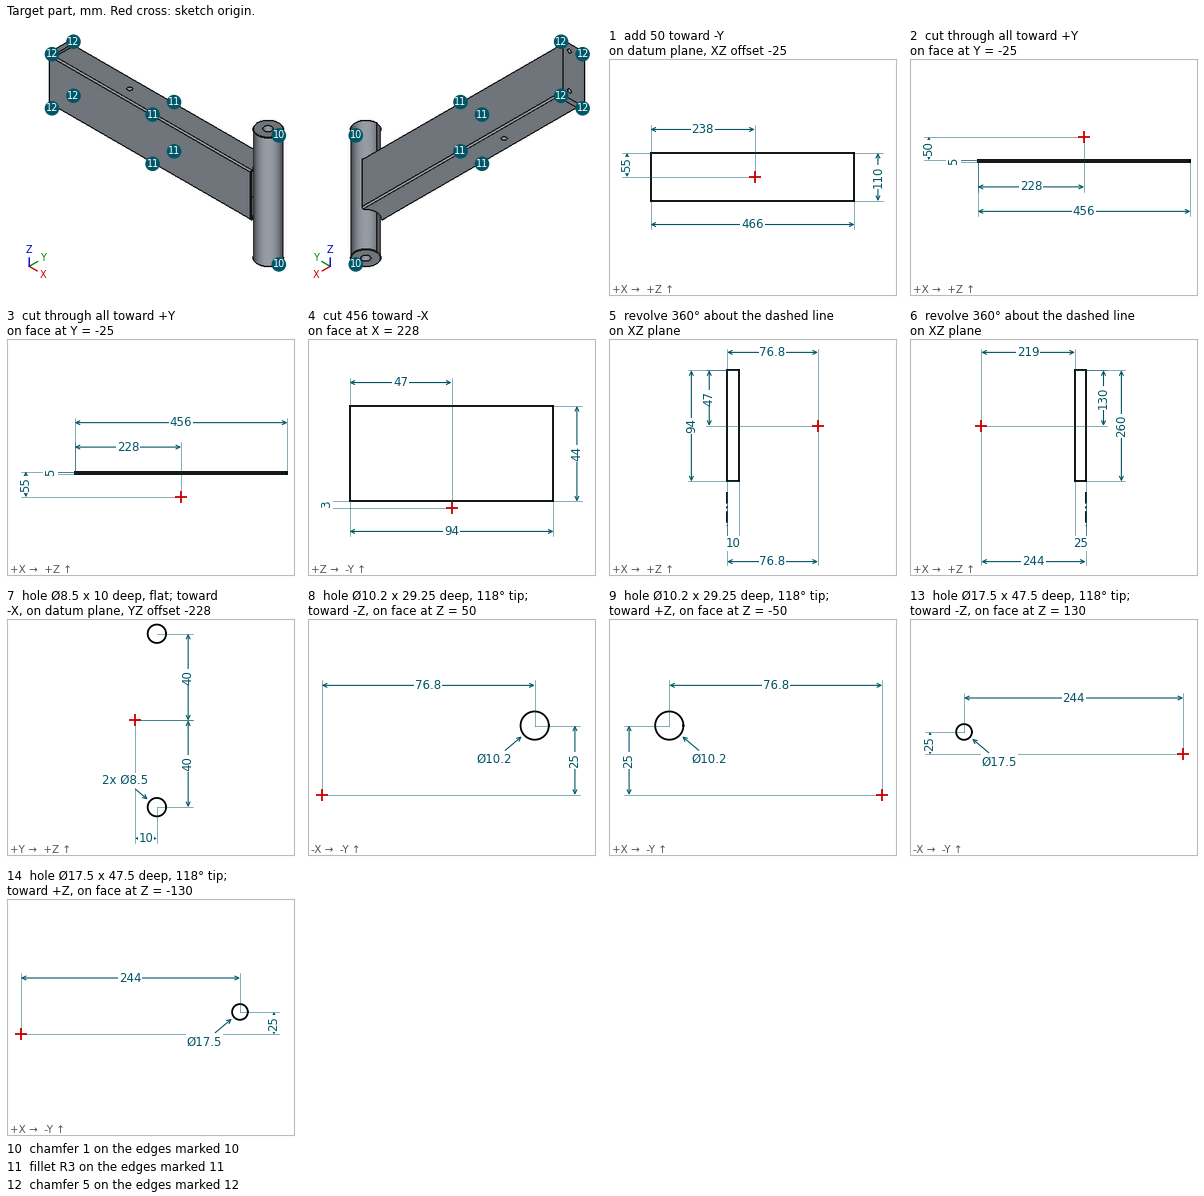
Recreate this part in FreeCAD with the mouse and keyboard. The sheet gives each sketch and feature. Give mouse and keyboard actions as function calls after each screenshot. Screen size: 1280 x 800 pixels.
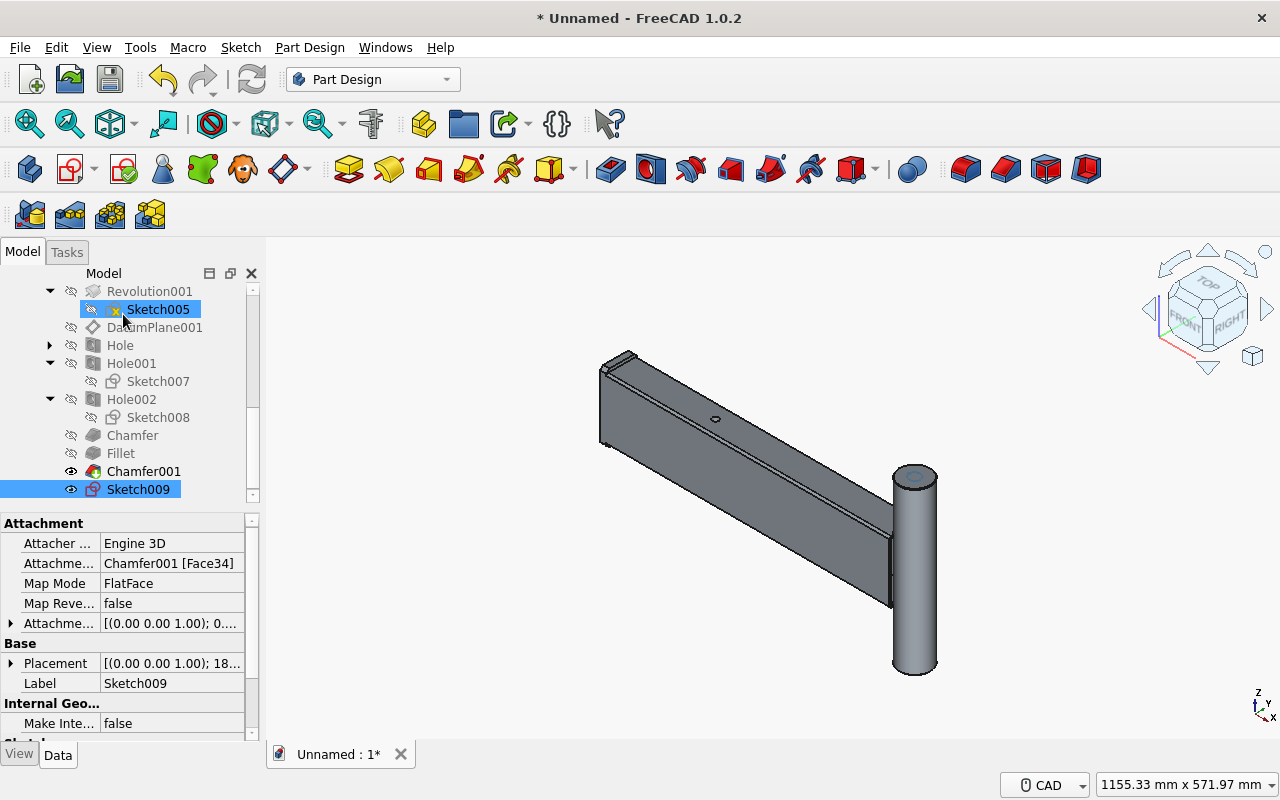
click(652, 170)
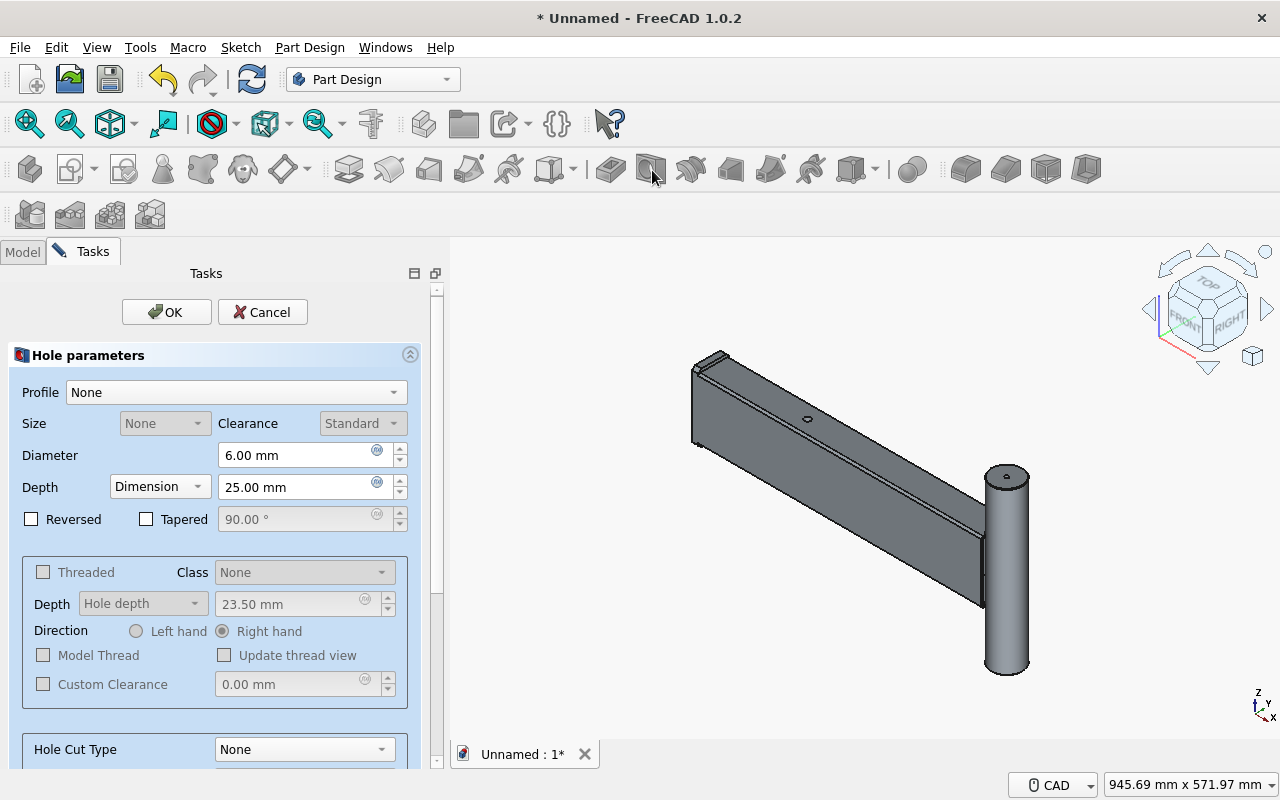
triple_click(305, 455)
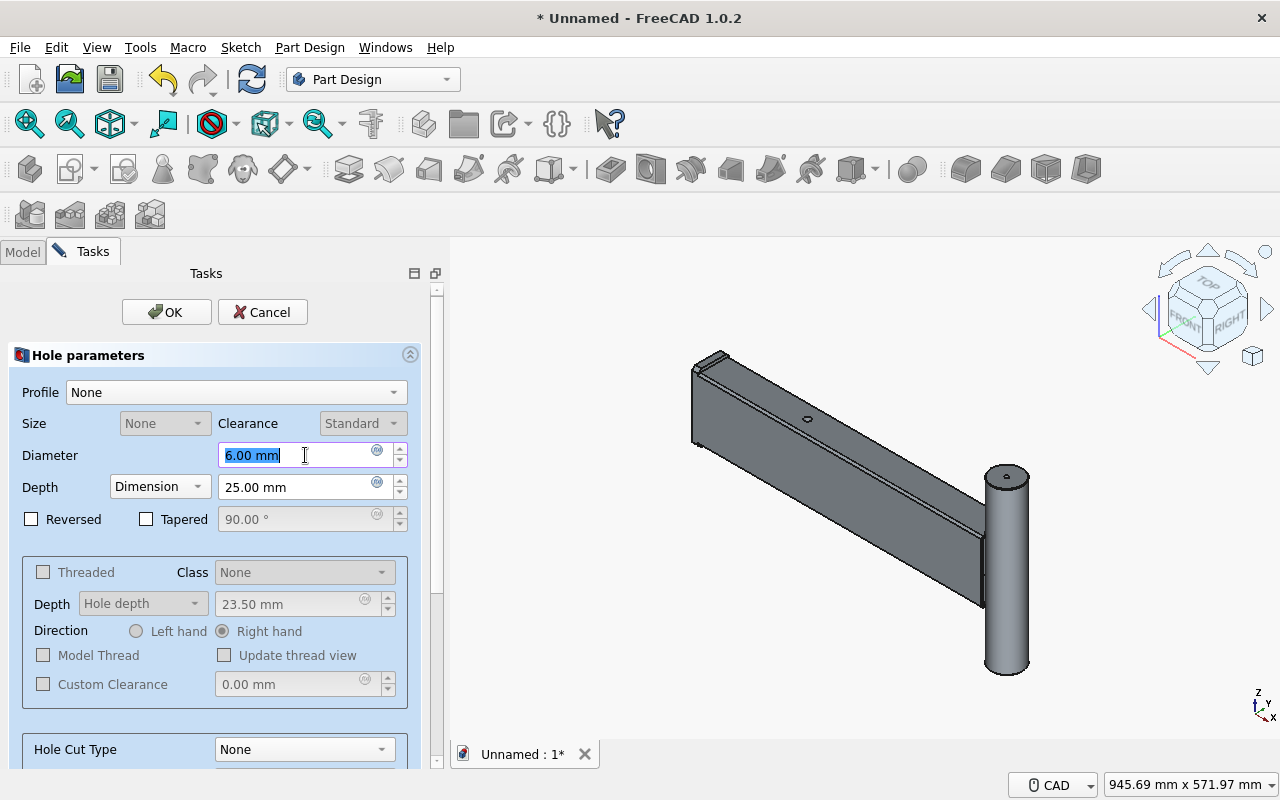
text(17.5)
key(Tab)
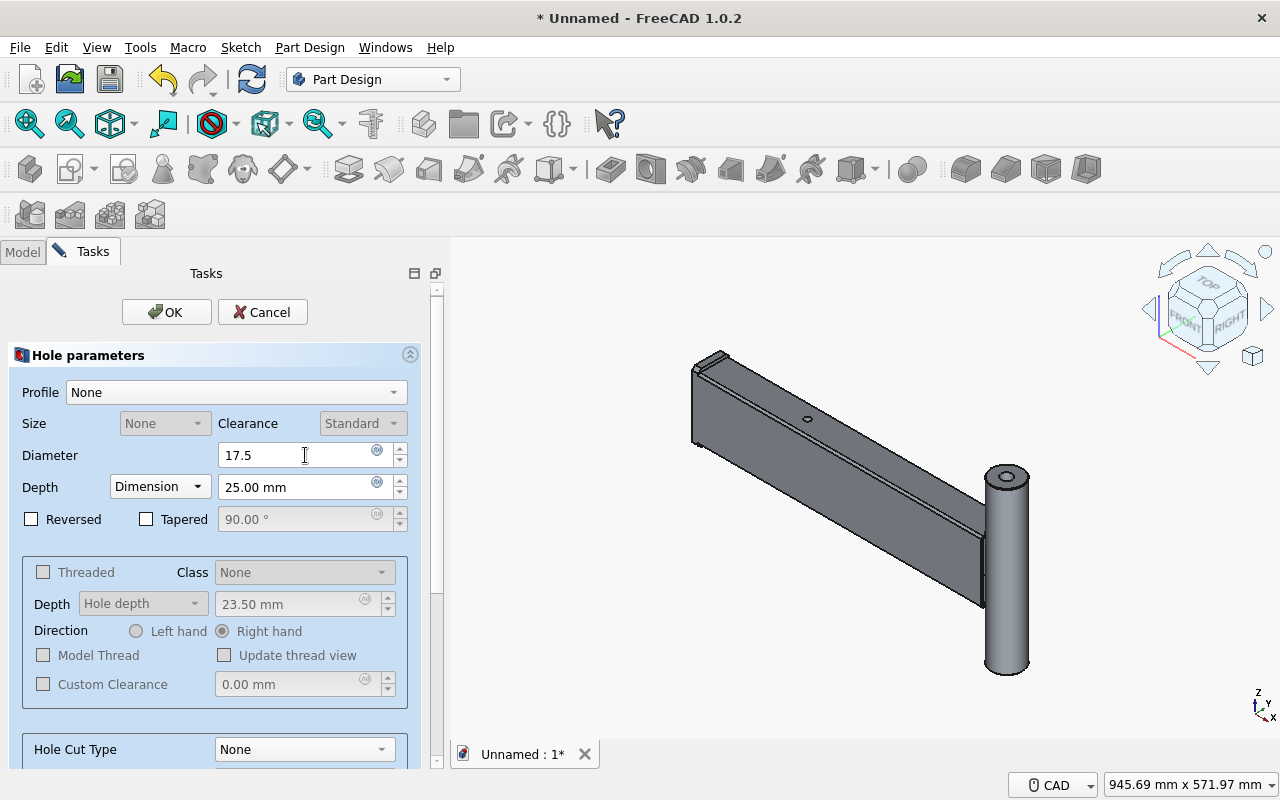
triple_click(305, 487)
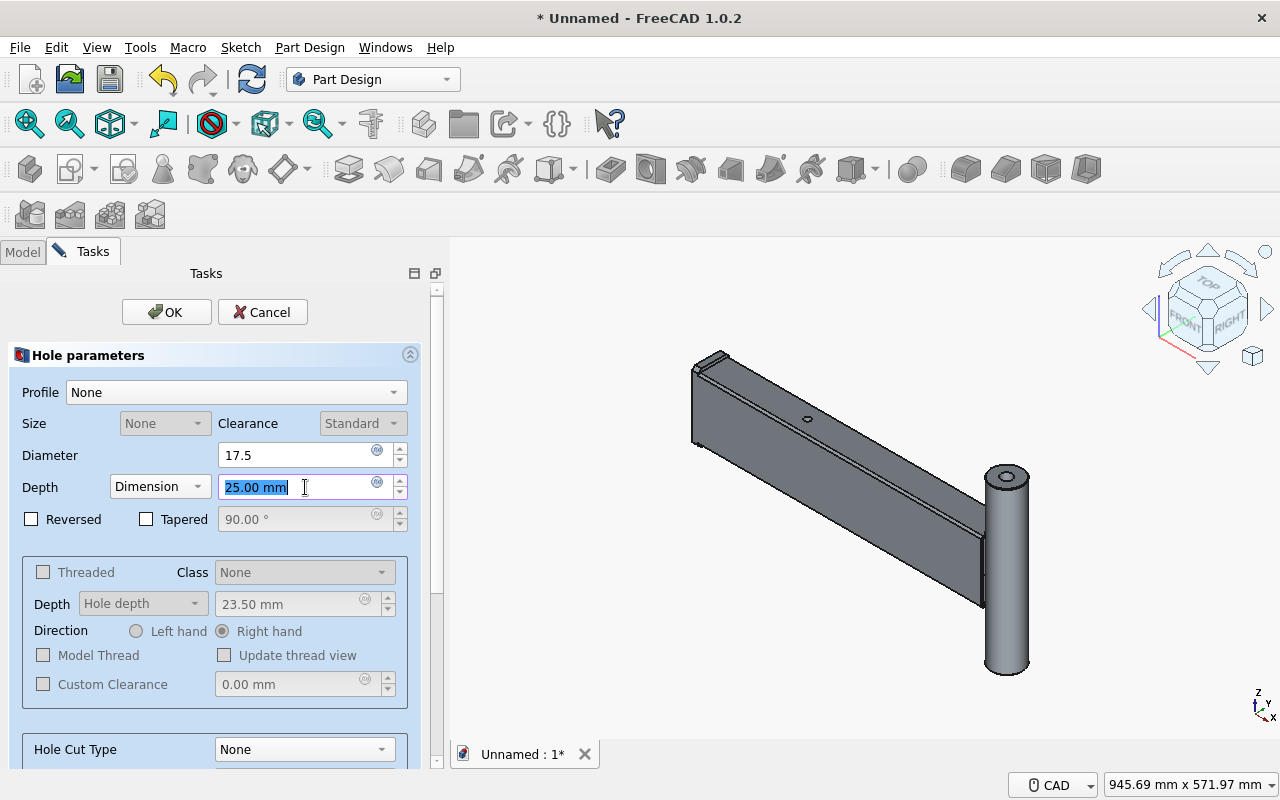
text(47.5)
key(Tab)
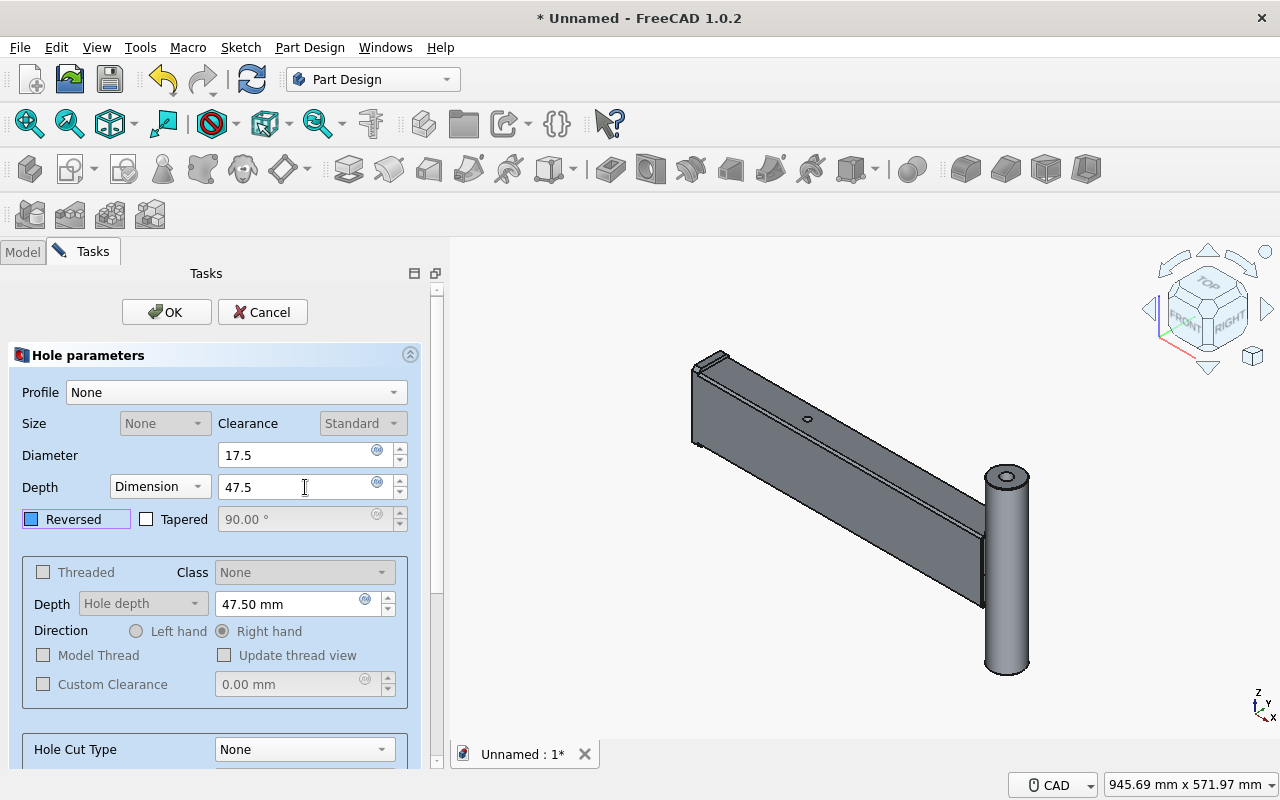
click(167, 312)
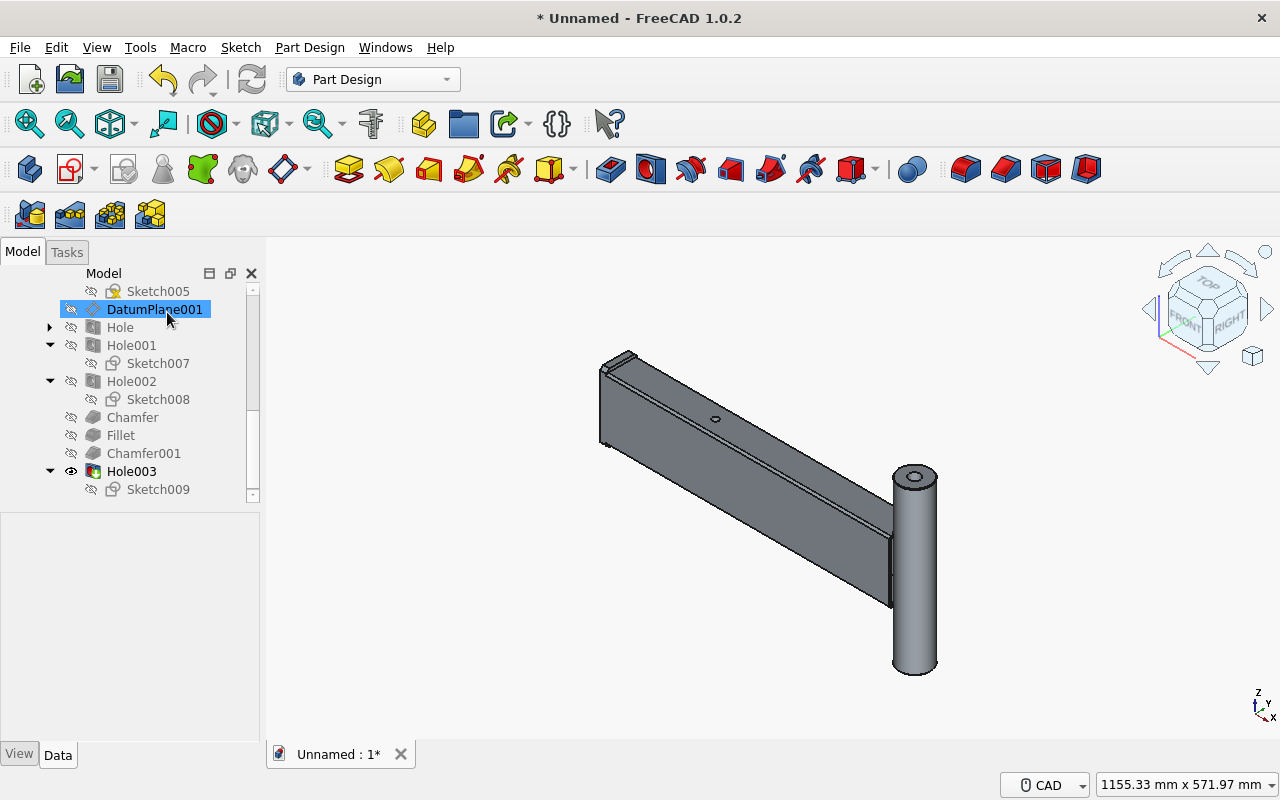
key(5)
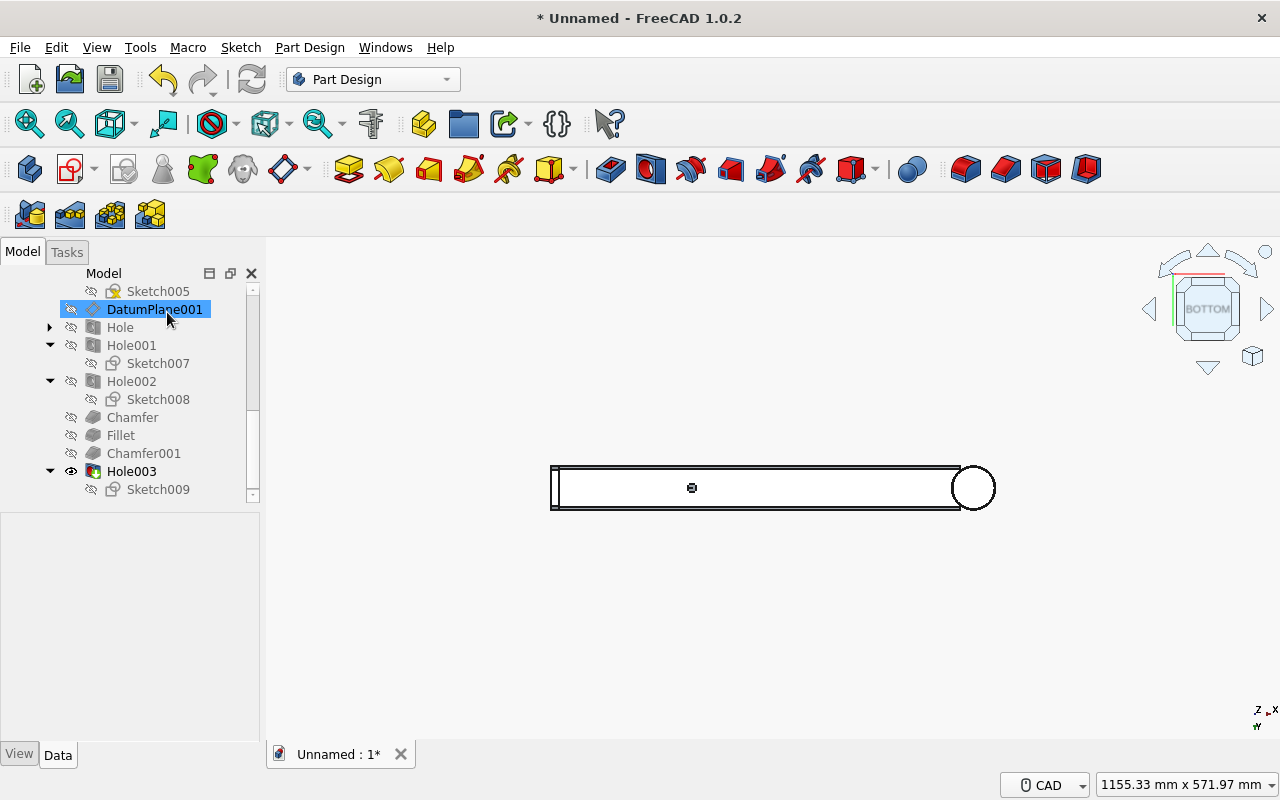
click(30, 124)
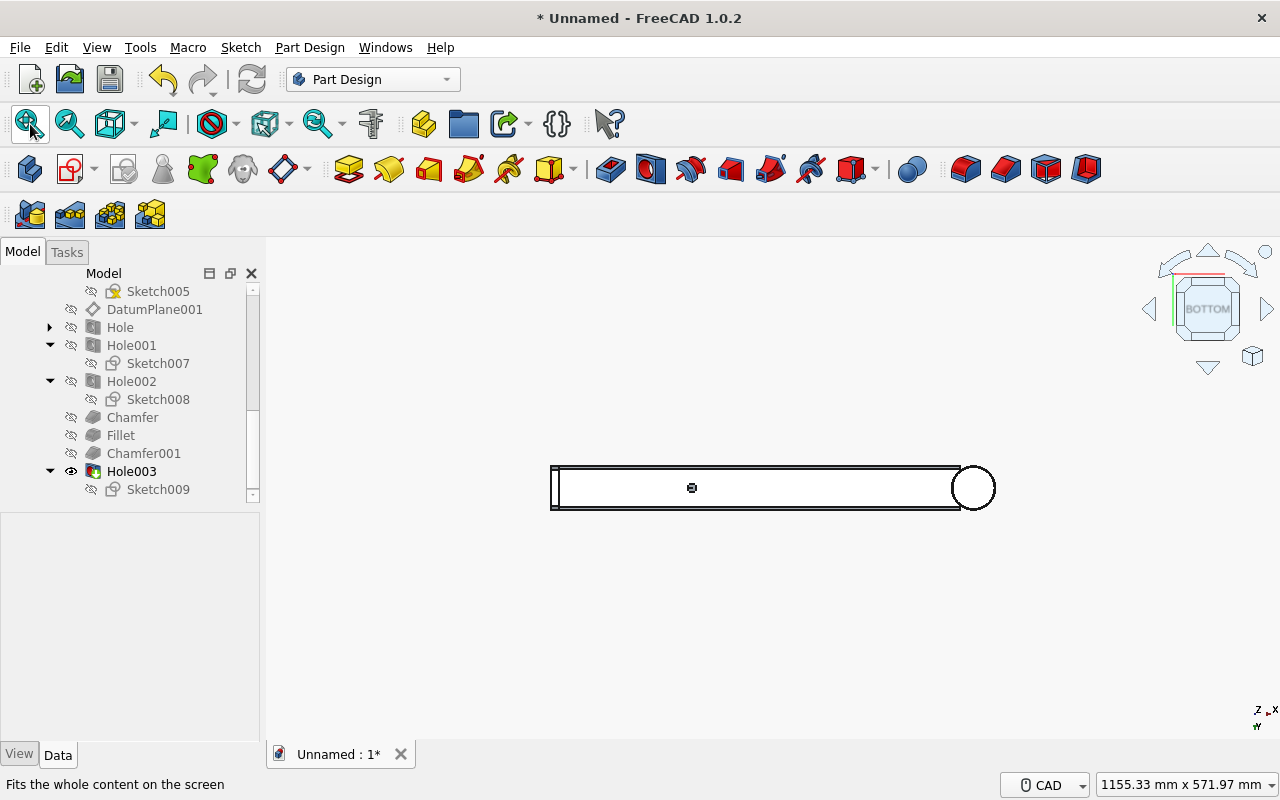
click(974, 487)